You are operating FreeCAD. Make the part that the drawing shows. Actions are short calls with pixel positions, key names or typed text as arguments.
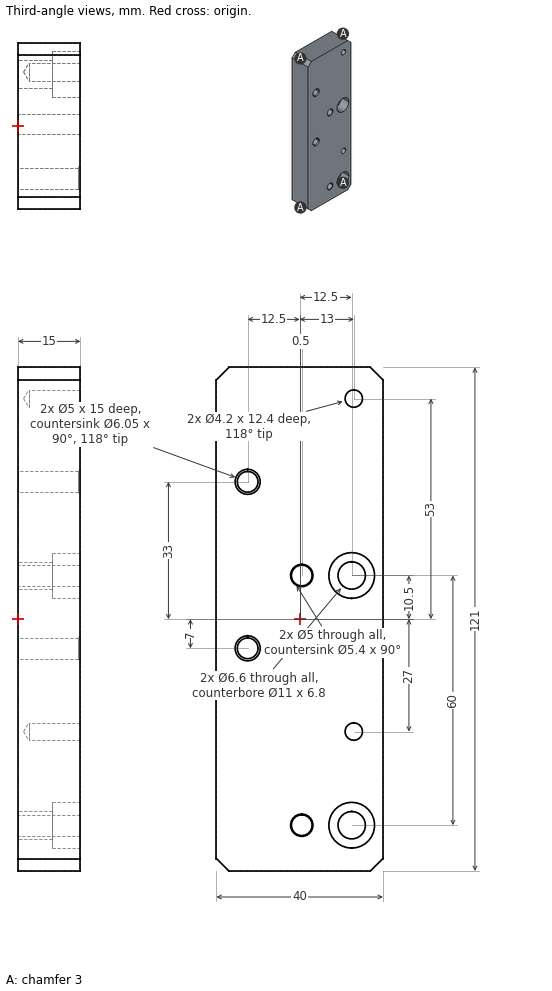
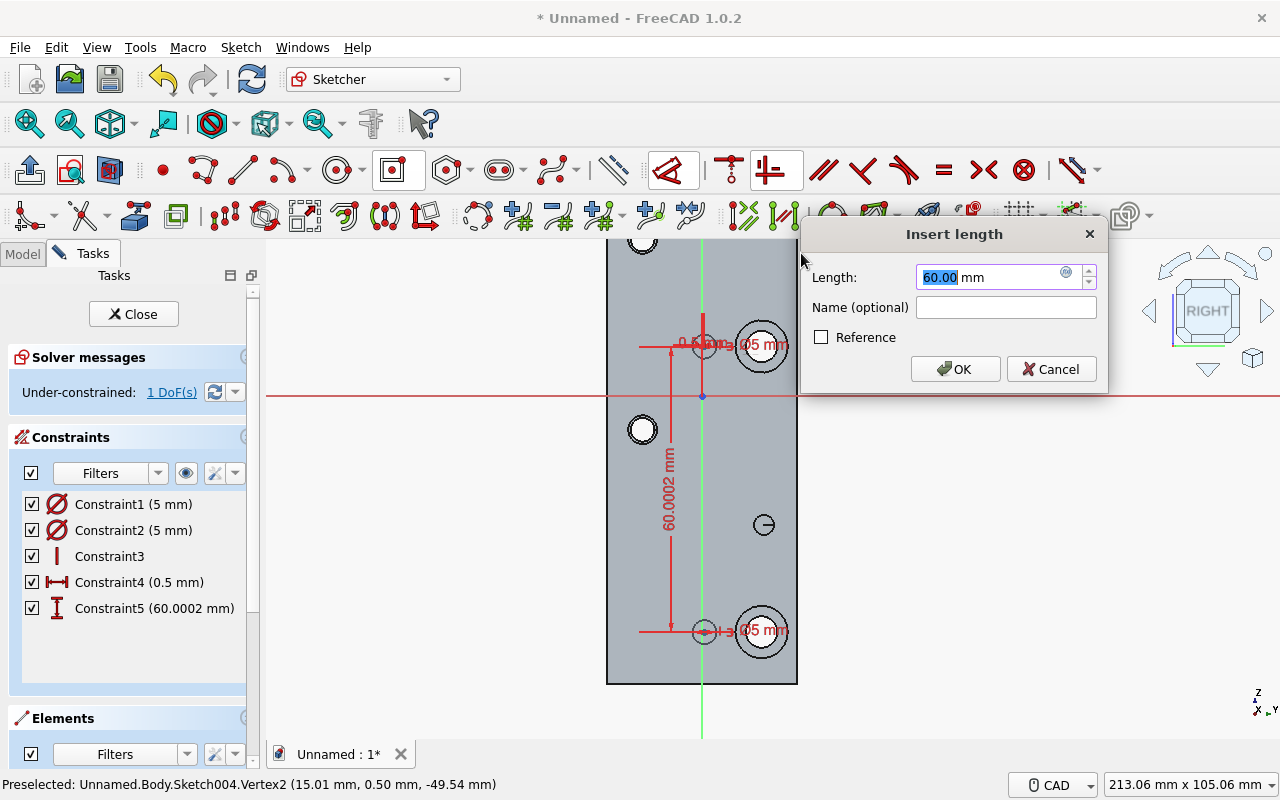
text(60)
key(Return)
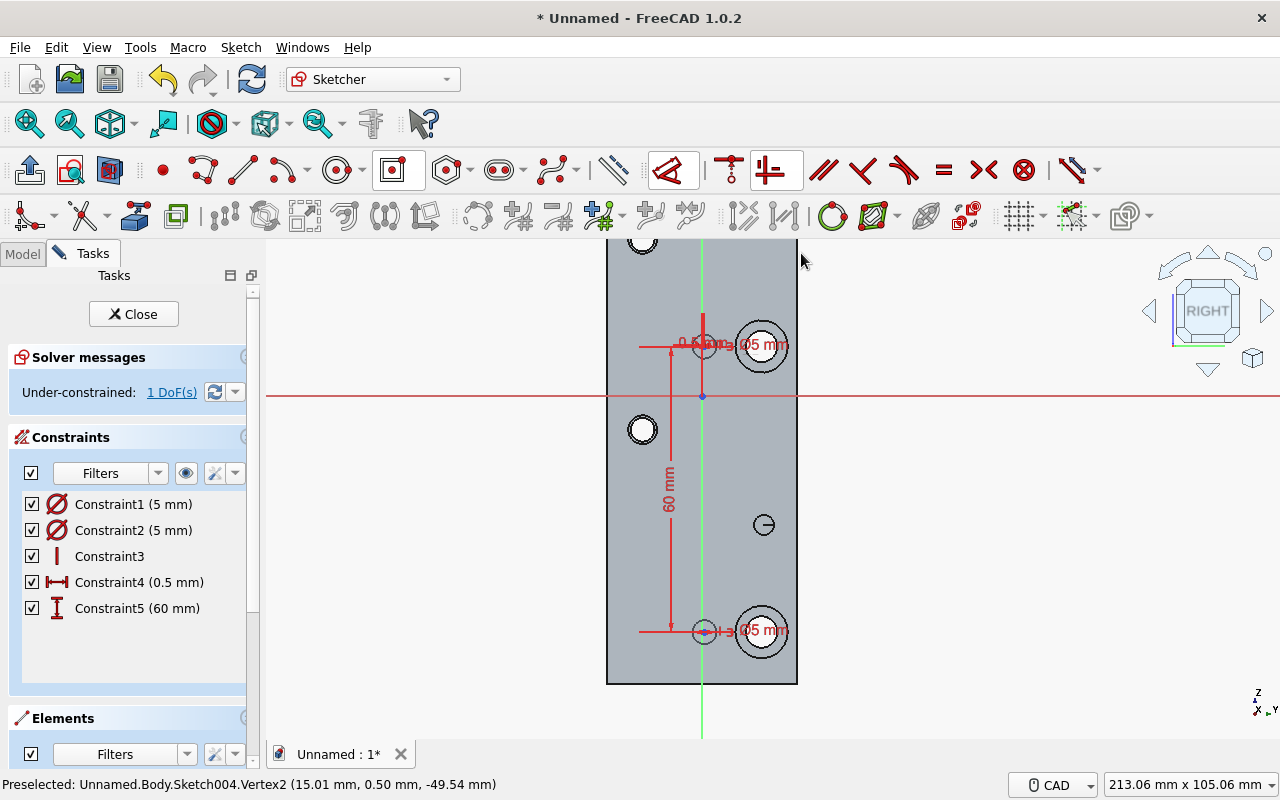
click(704, 347)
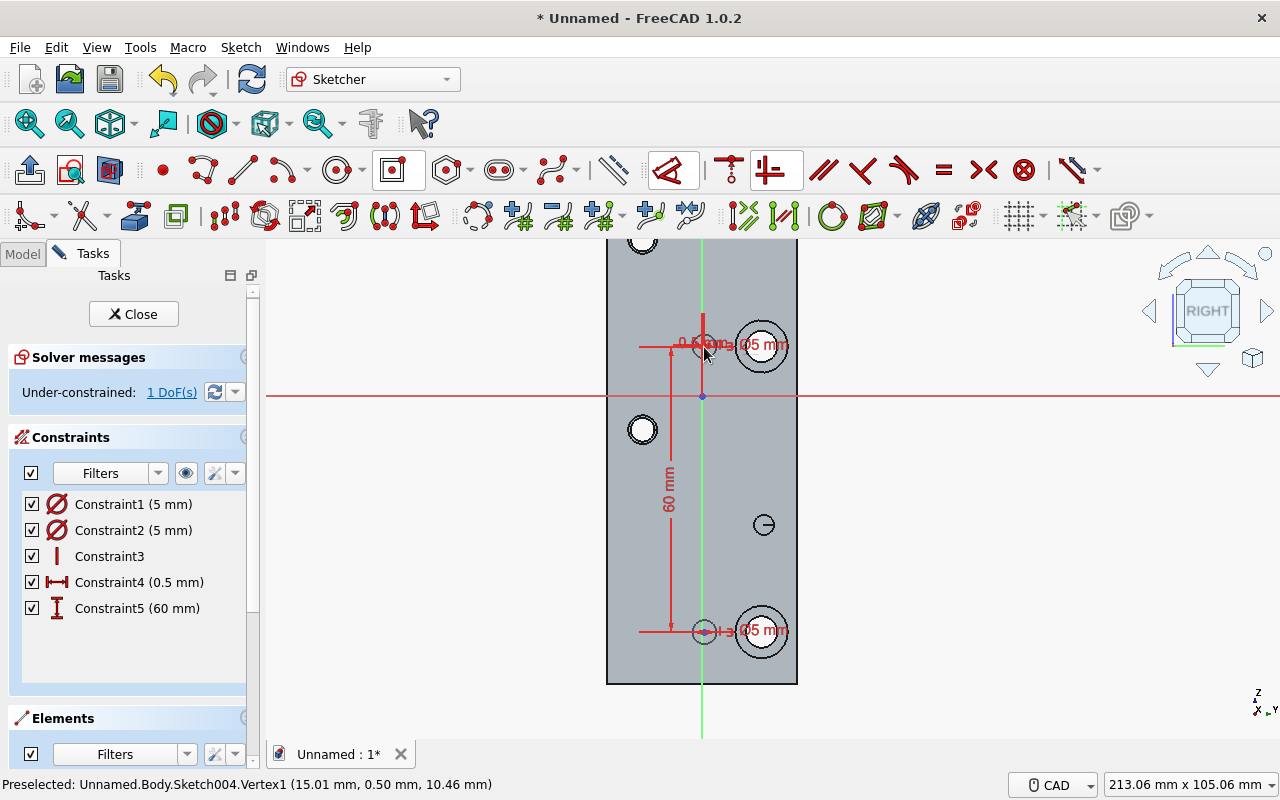
click(694, 170)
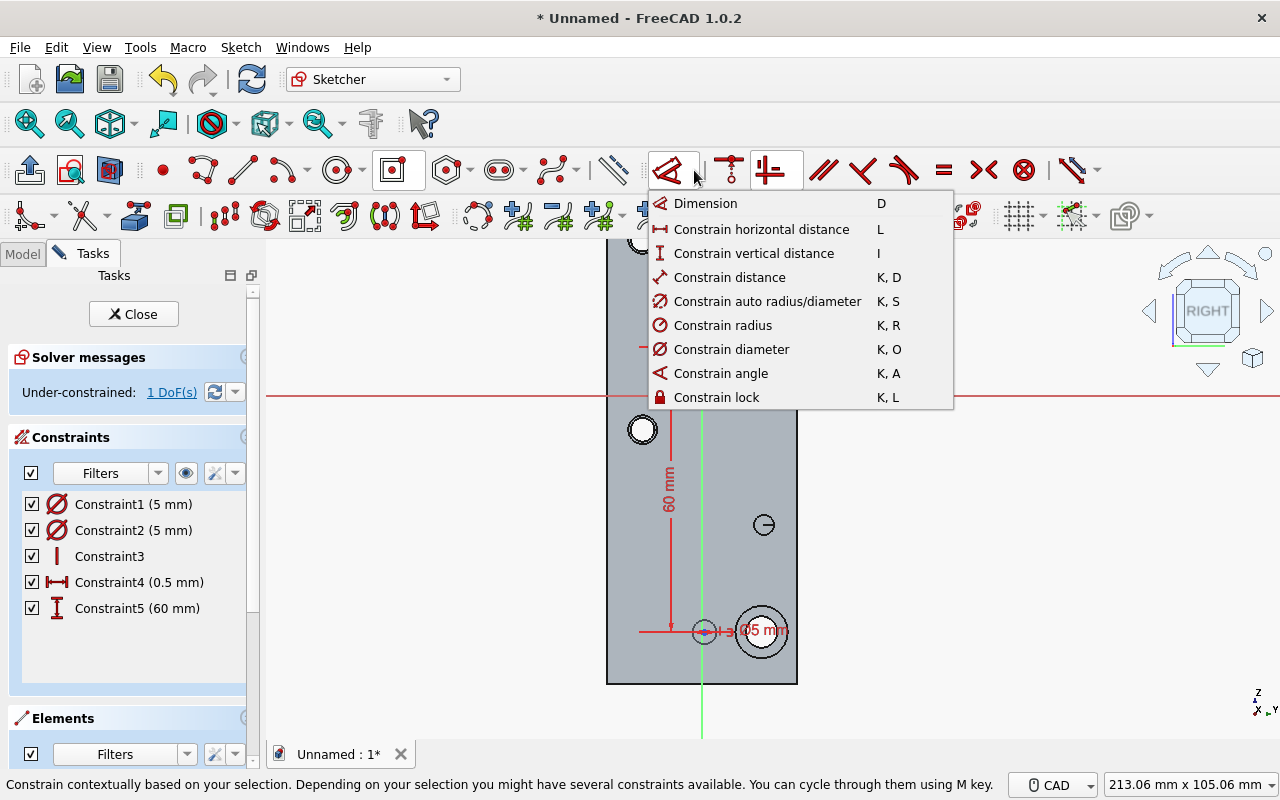
click(801, 253)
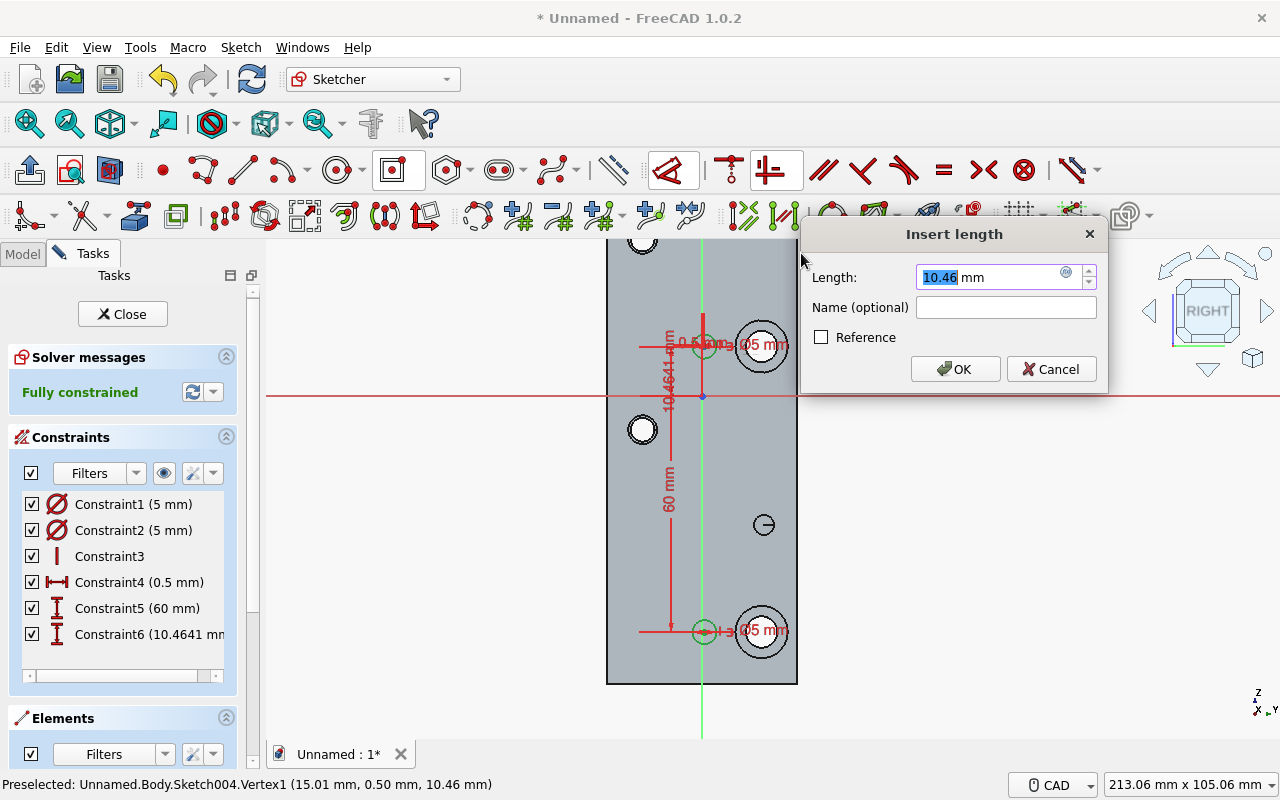
text(10.5)
key(Return)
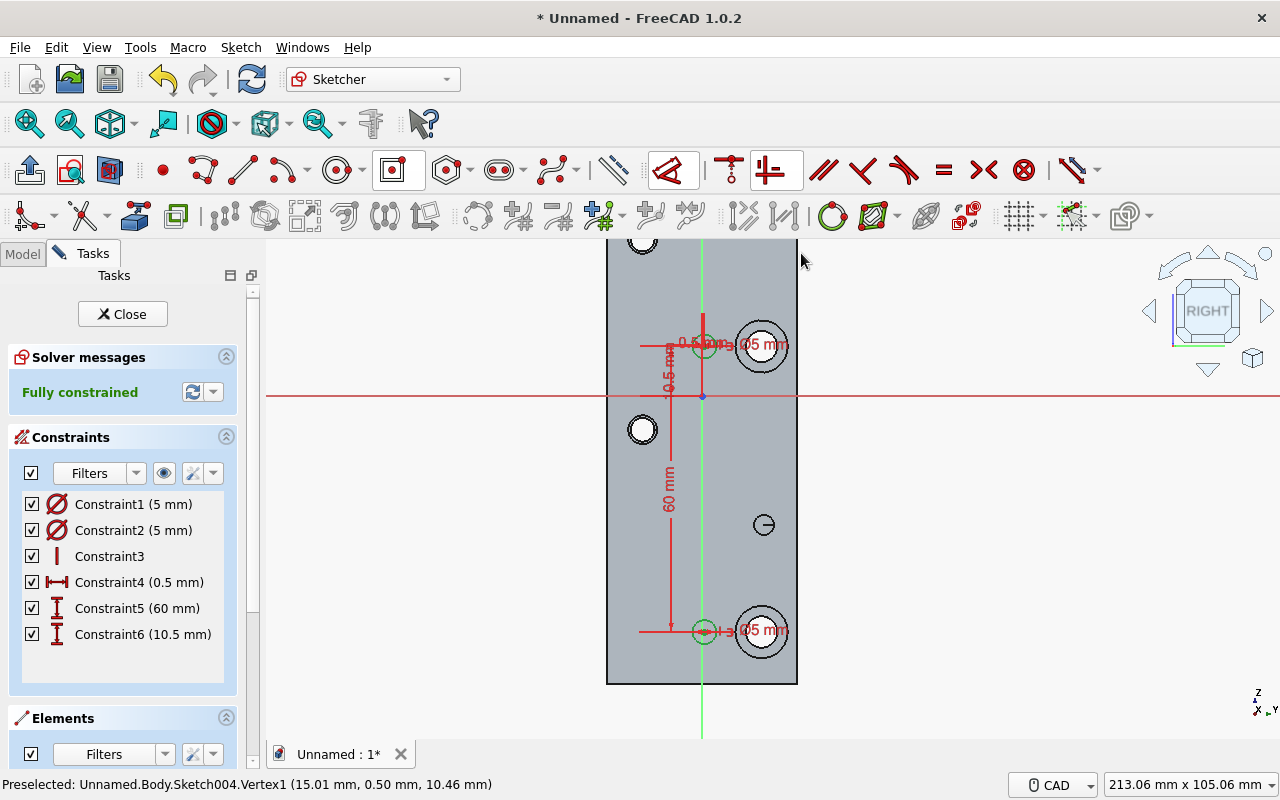
click(123, 314)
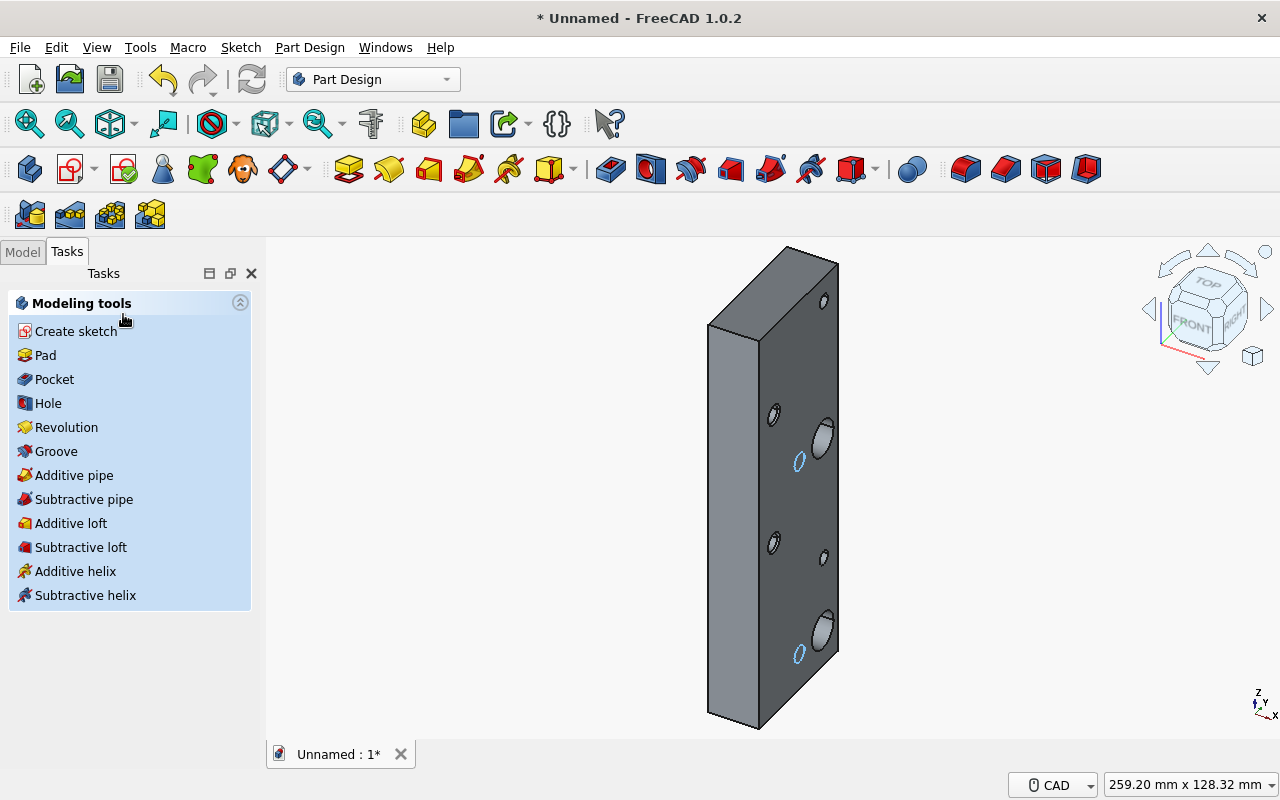
click(652, 170)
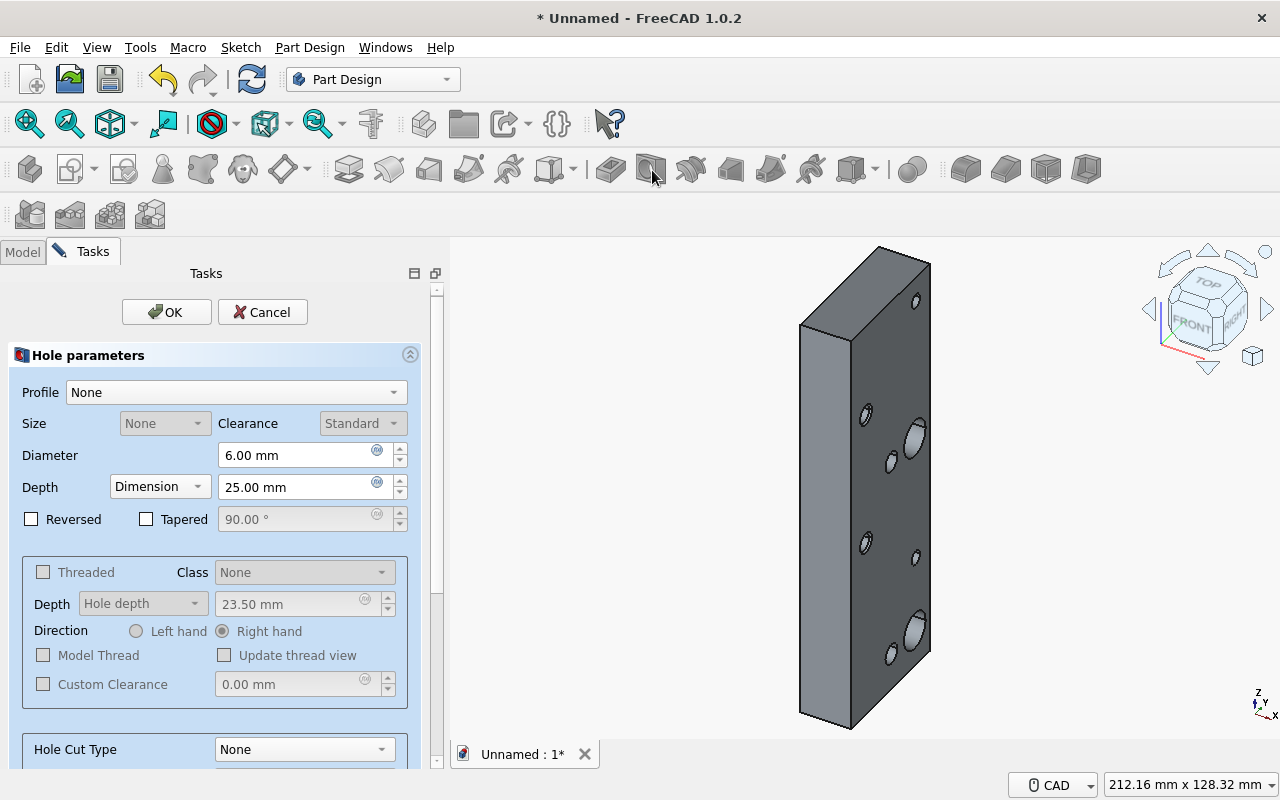
triple_click(305, 455)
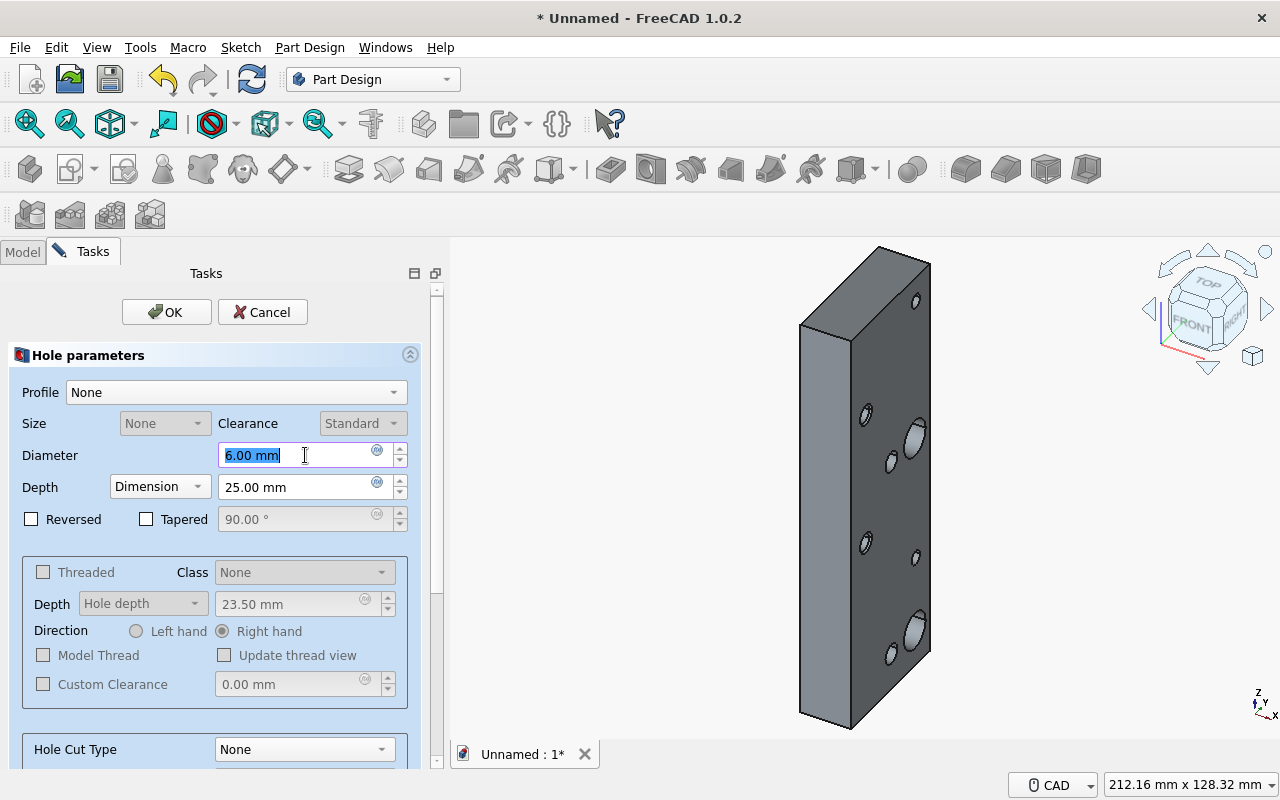
text(5)
key(Tab)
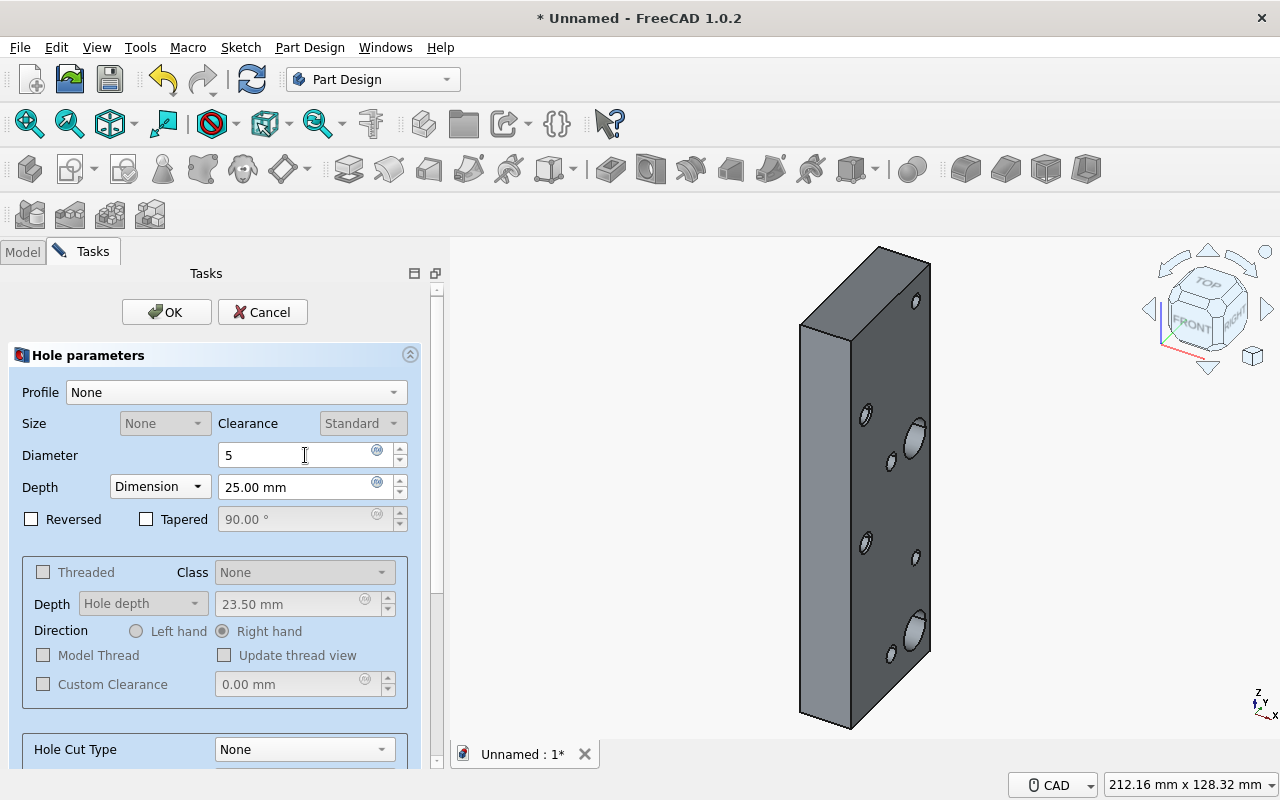
click(161, 486)